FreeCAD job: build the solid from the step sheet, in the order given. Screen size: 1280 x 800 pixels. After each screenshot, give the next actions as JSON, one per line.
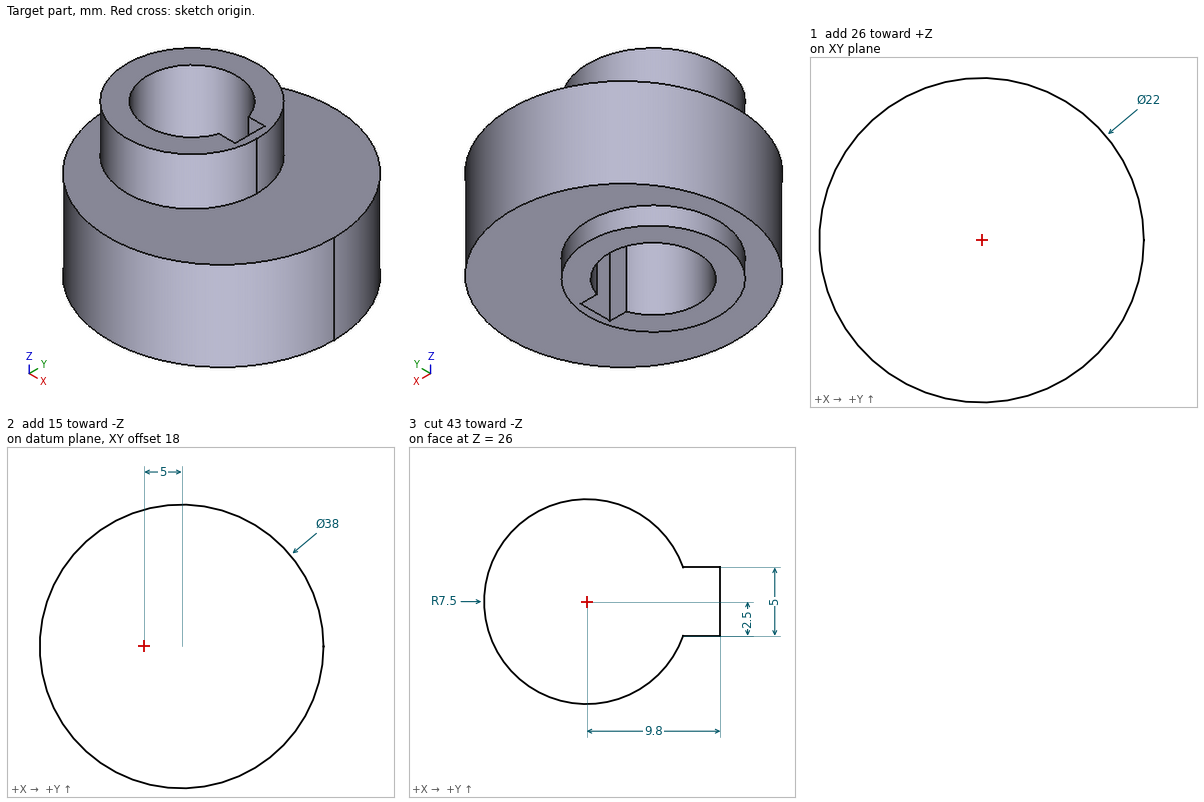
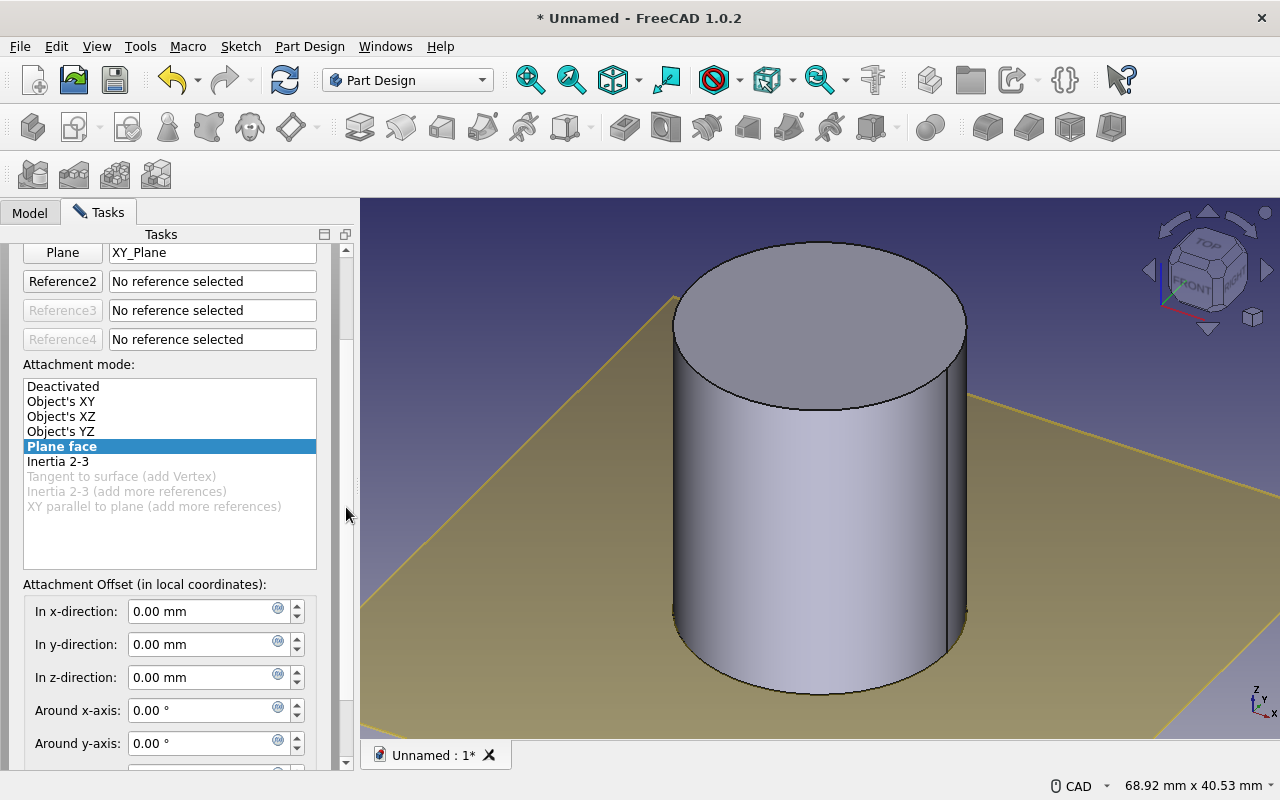
{"action": "triple_click", "coordinate": [210, 678]}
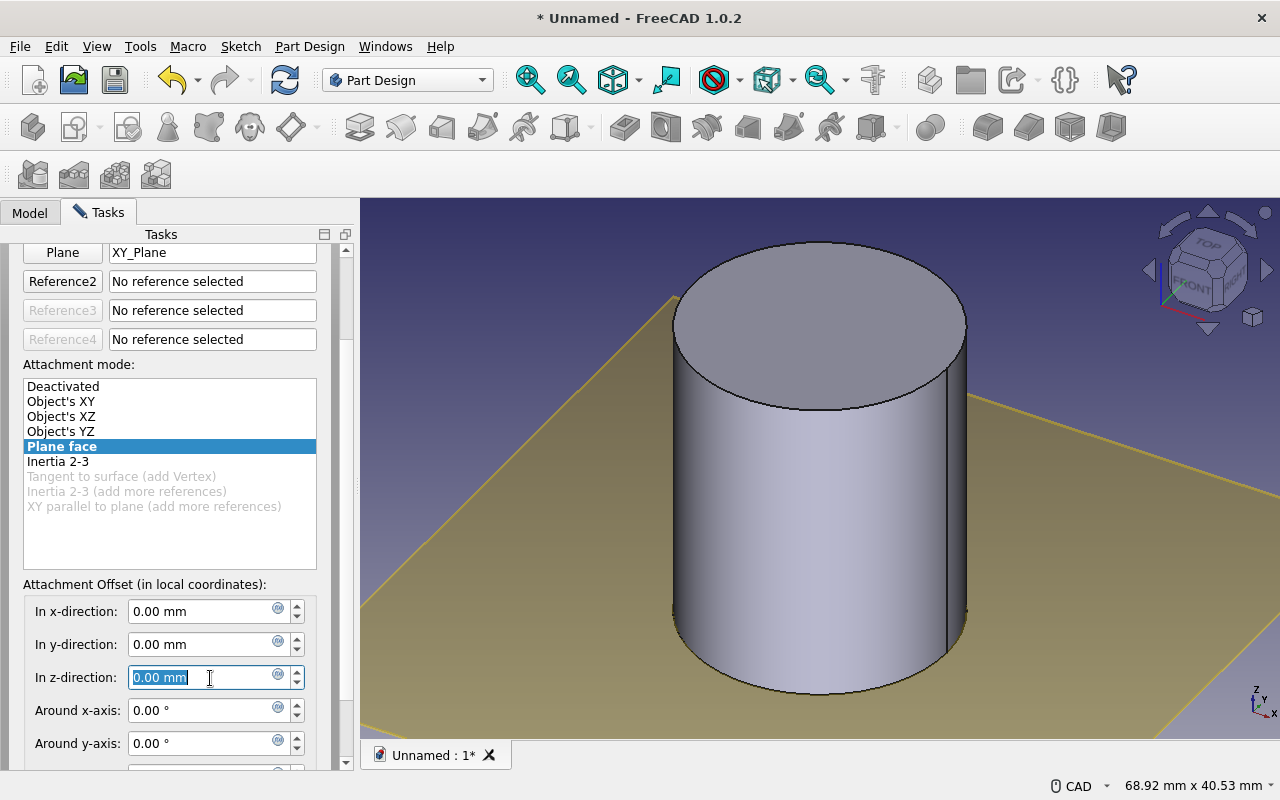
{"action": "type", "text": "18"}
{"action": "key", "text": "Tab"}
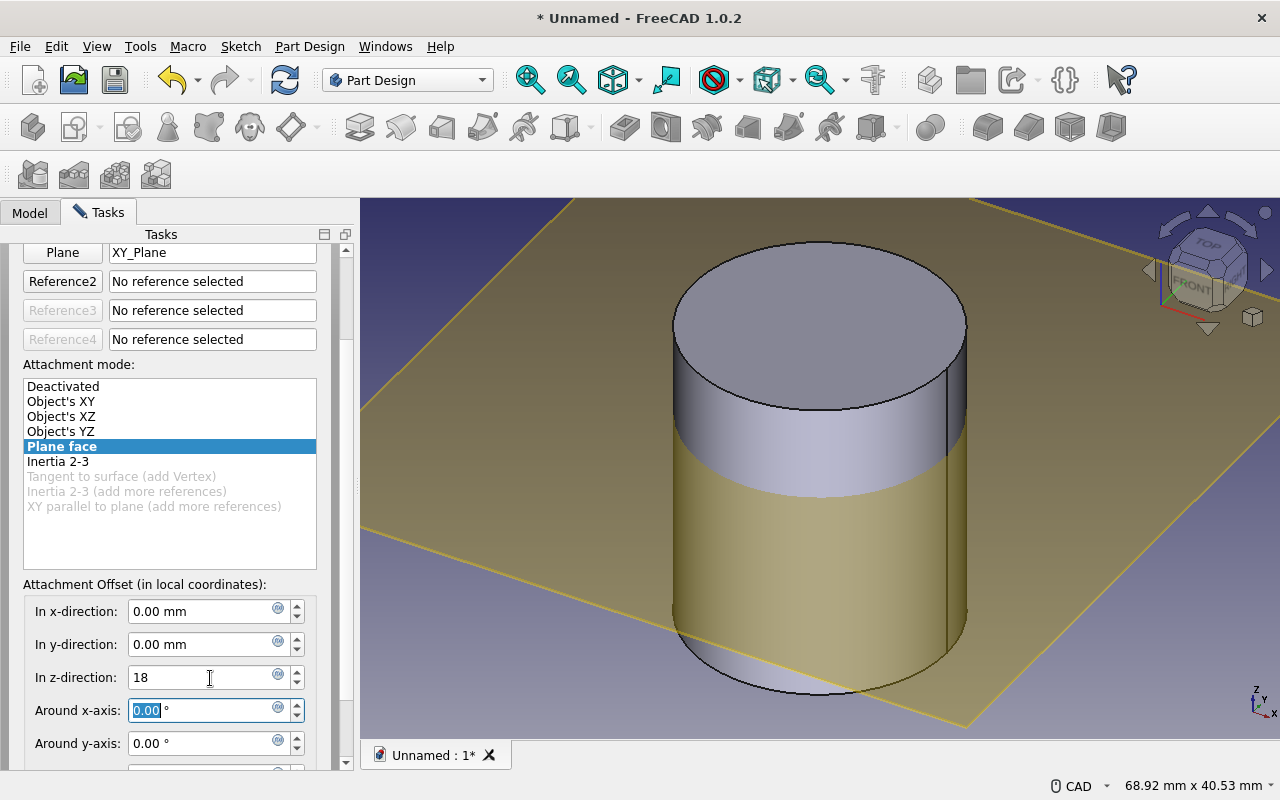
{"action": "scroll", "coordinate": [346, 507], "scroll_direction": "up", "scroll_amount": 3}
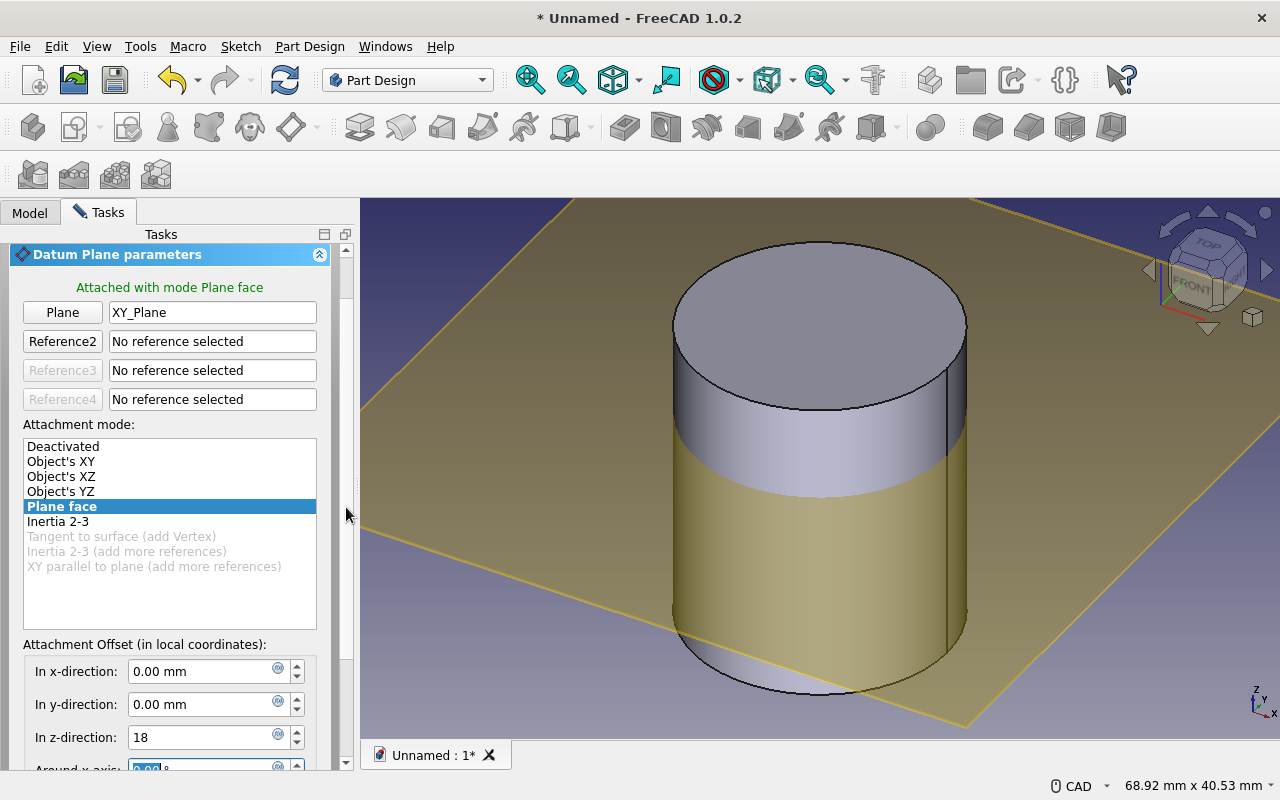
{"action": "left_click", "coordinate": [127, 273]}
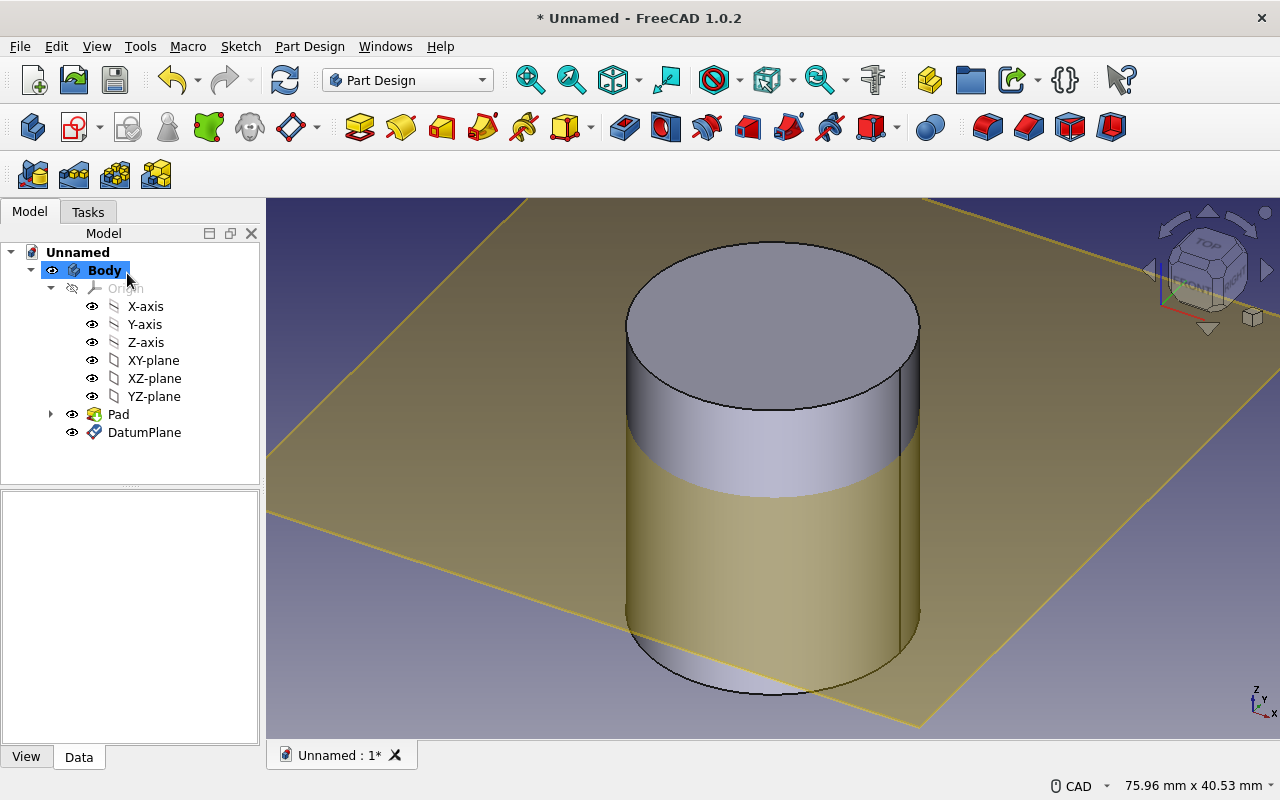
{"action": "left_click", "coordinate": [117, 432]}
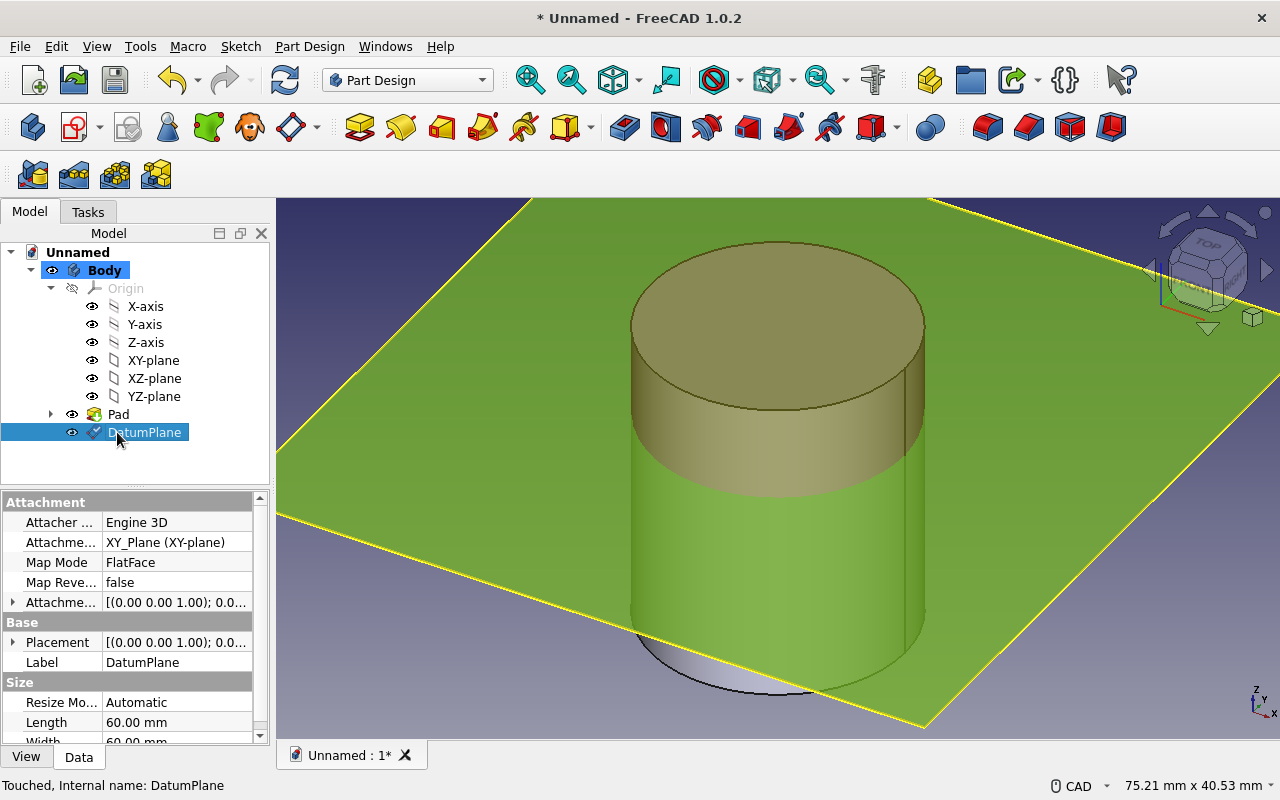
{"action": "left_click", "coordinate": [74, 128]}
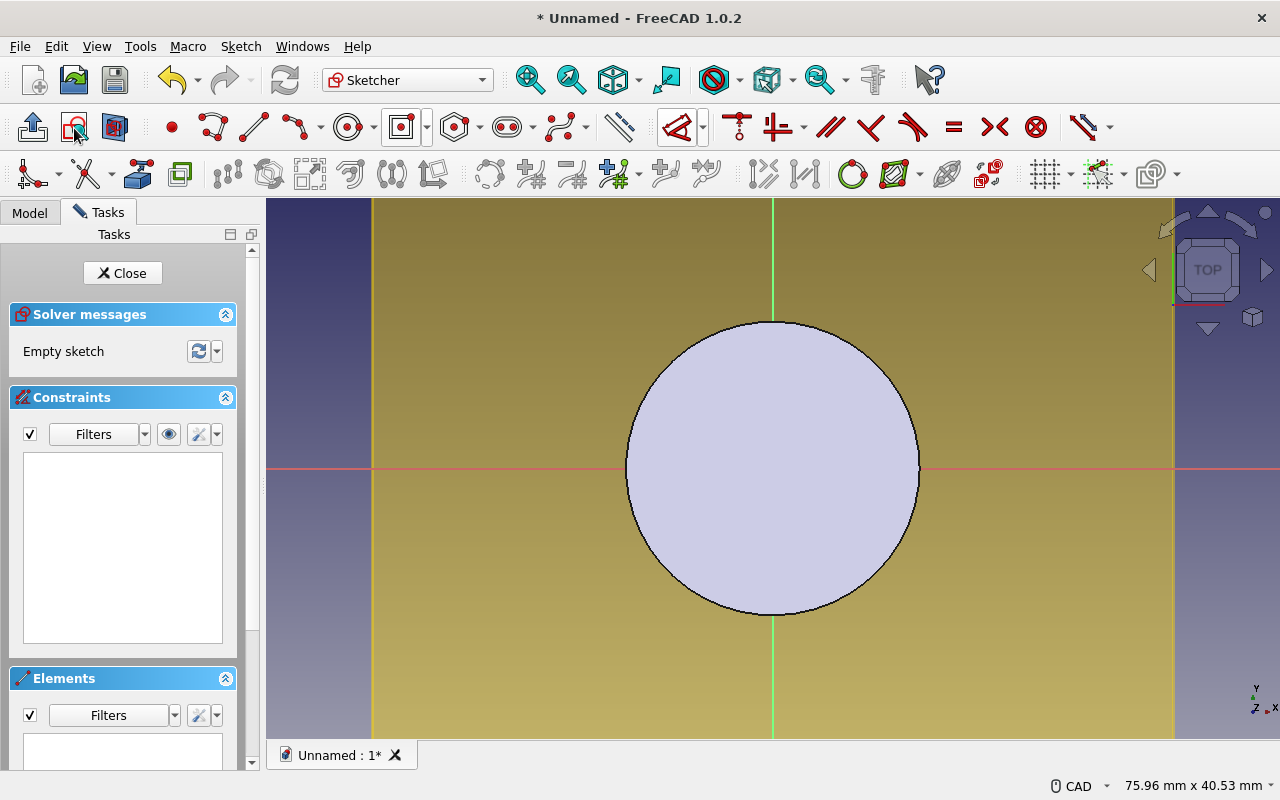
{"action": "left_click", "coordinate": [115, 128]}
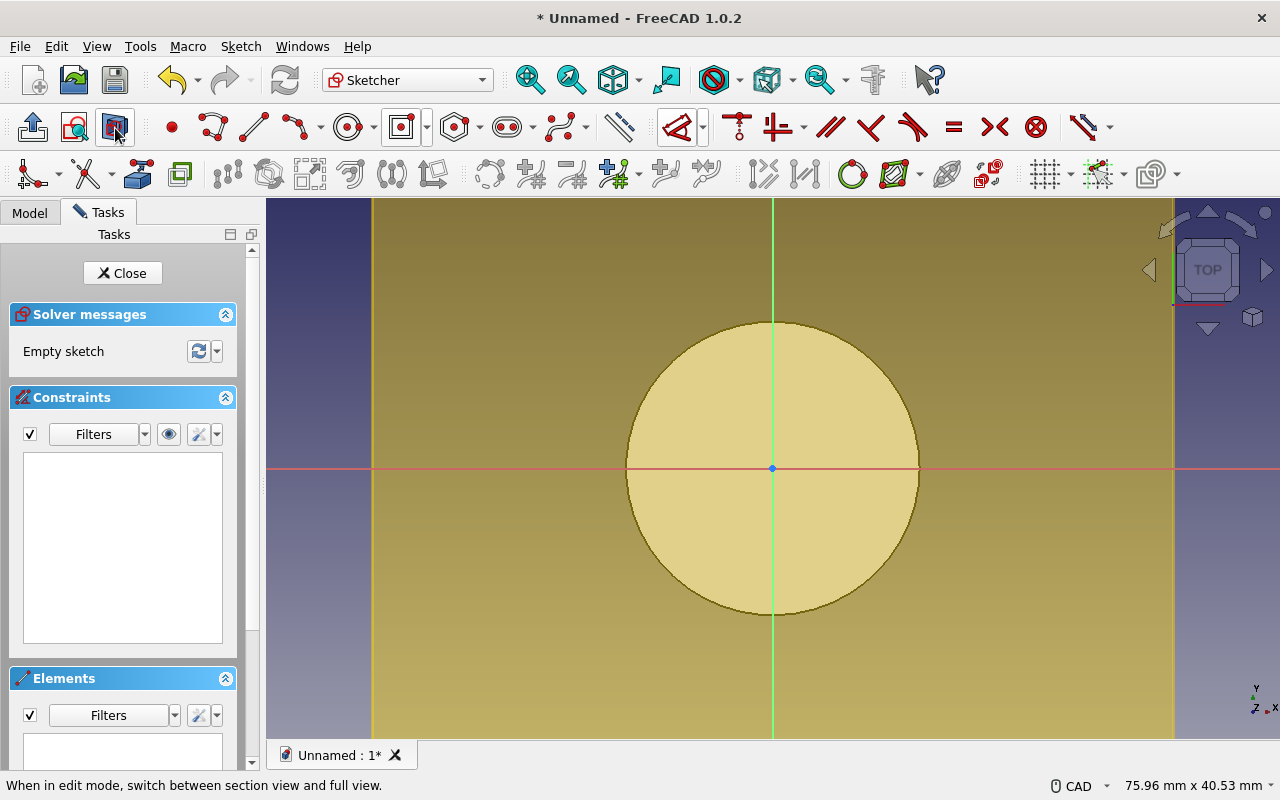
{"action": "scroll", "coordinate": [430, 468], "scroll_direction": "down", "scroll_amount": 2}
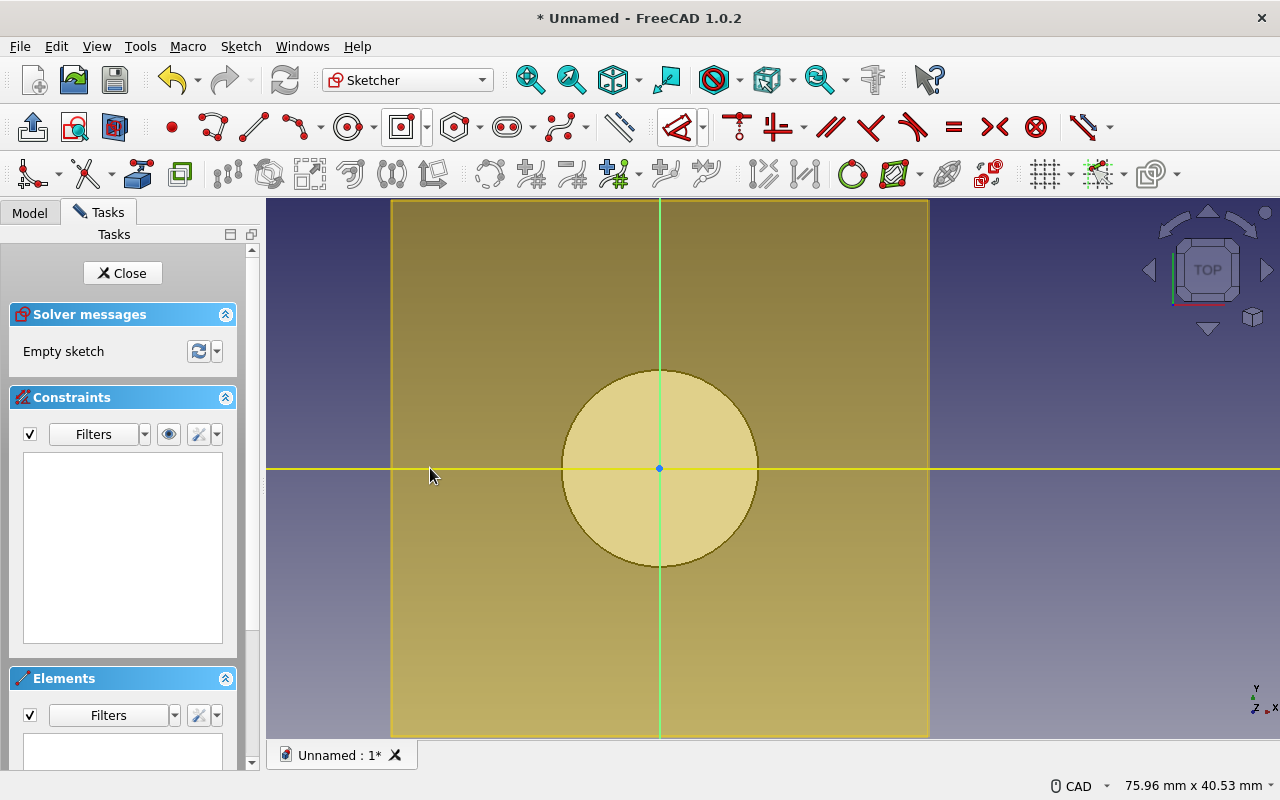
{"action": "key", "text": "g c"}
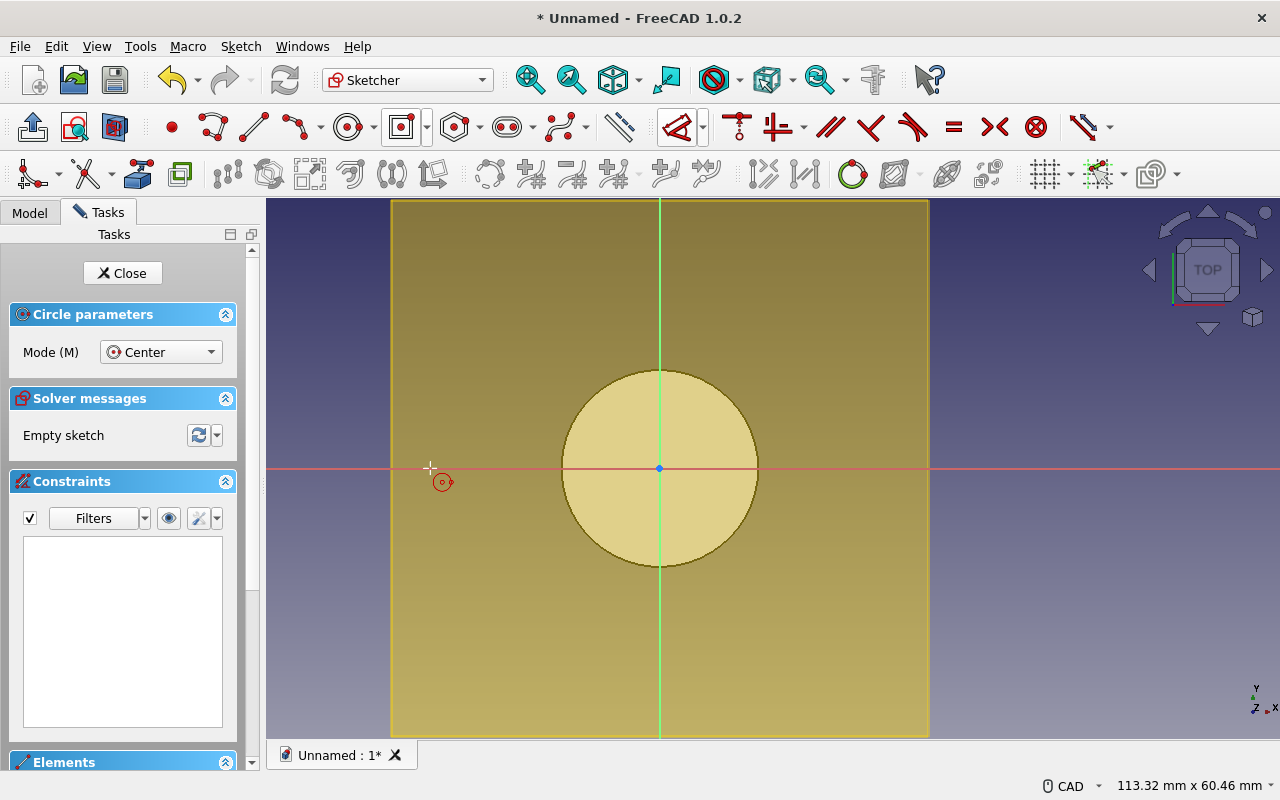
{"action": "left_click", "coordinate": [705, 468]}
{"action": "left_click", "coordinate": [825, 348]}
{"action": "key", "text": "Escape"}